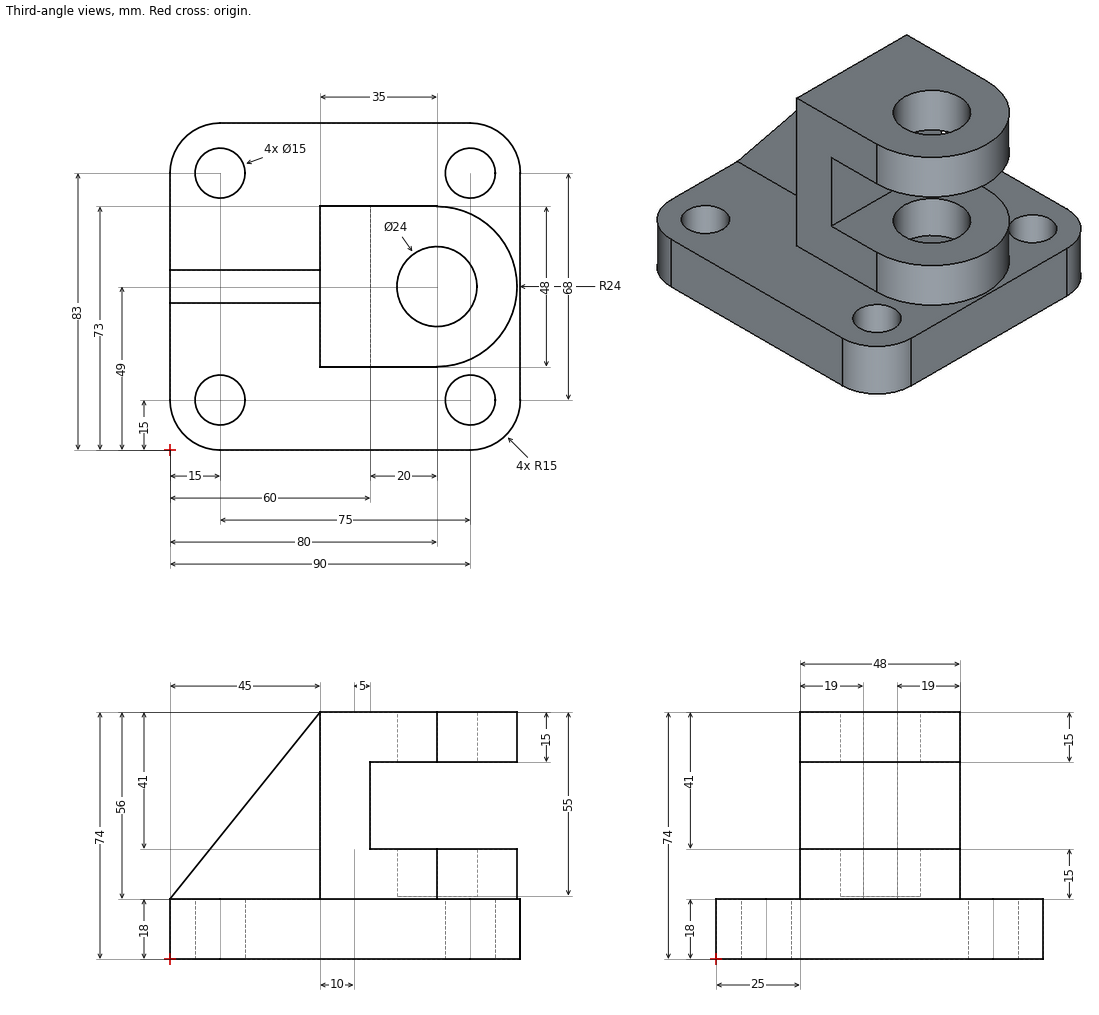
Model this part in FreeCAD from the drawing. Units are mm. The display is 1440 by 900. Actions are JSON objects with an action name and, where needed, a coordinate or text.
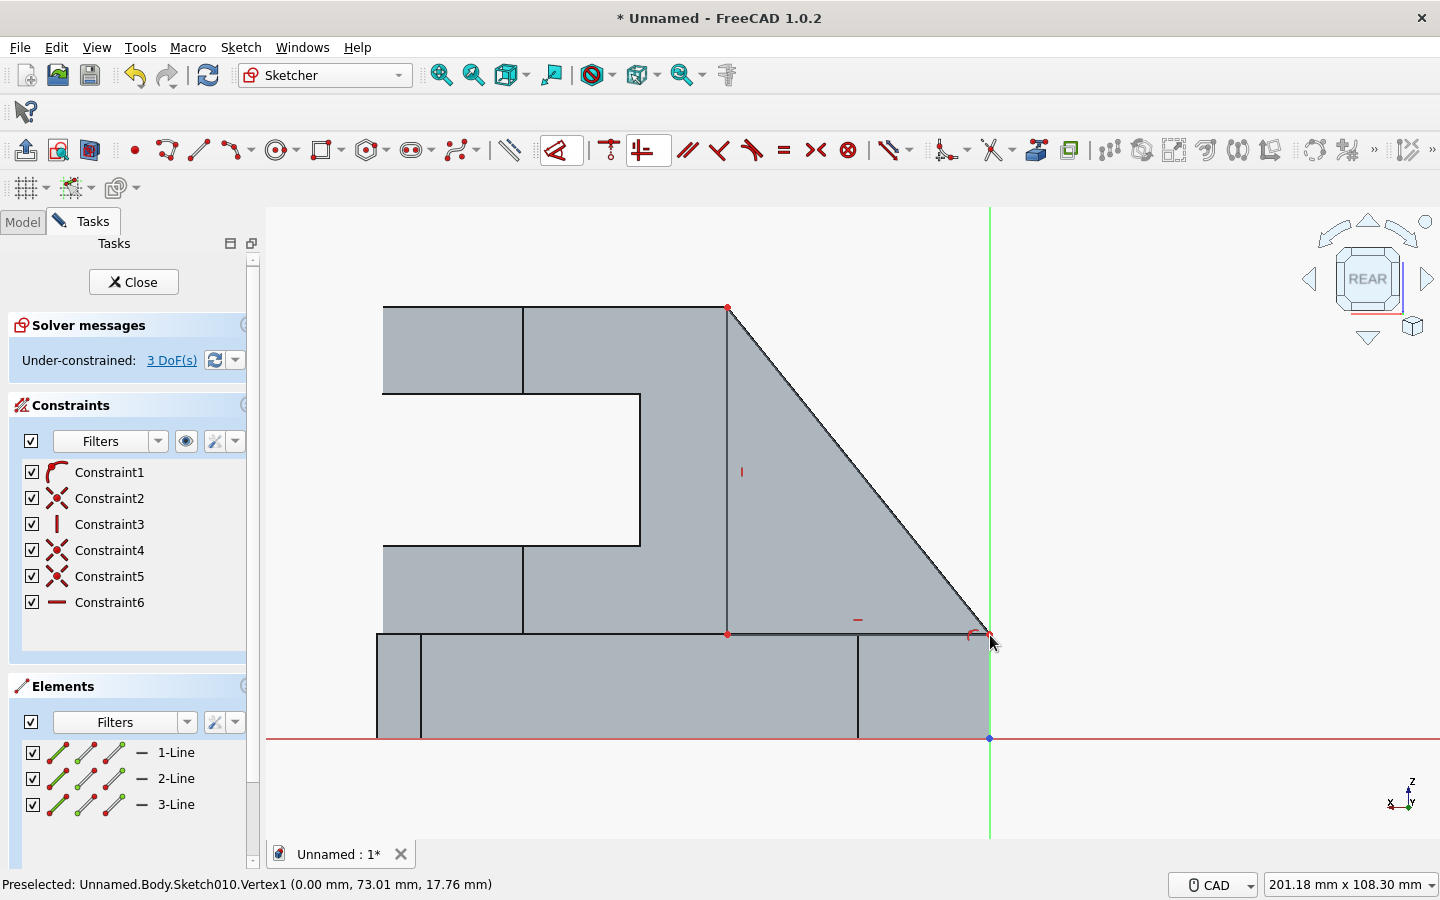
{"action": "left_click", "coordinate": [727, 406]}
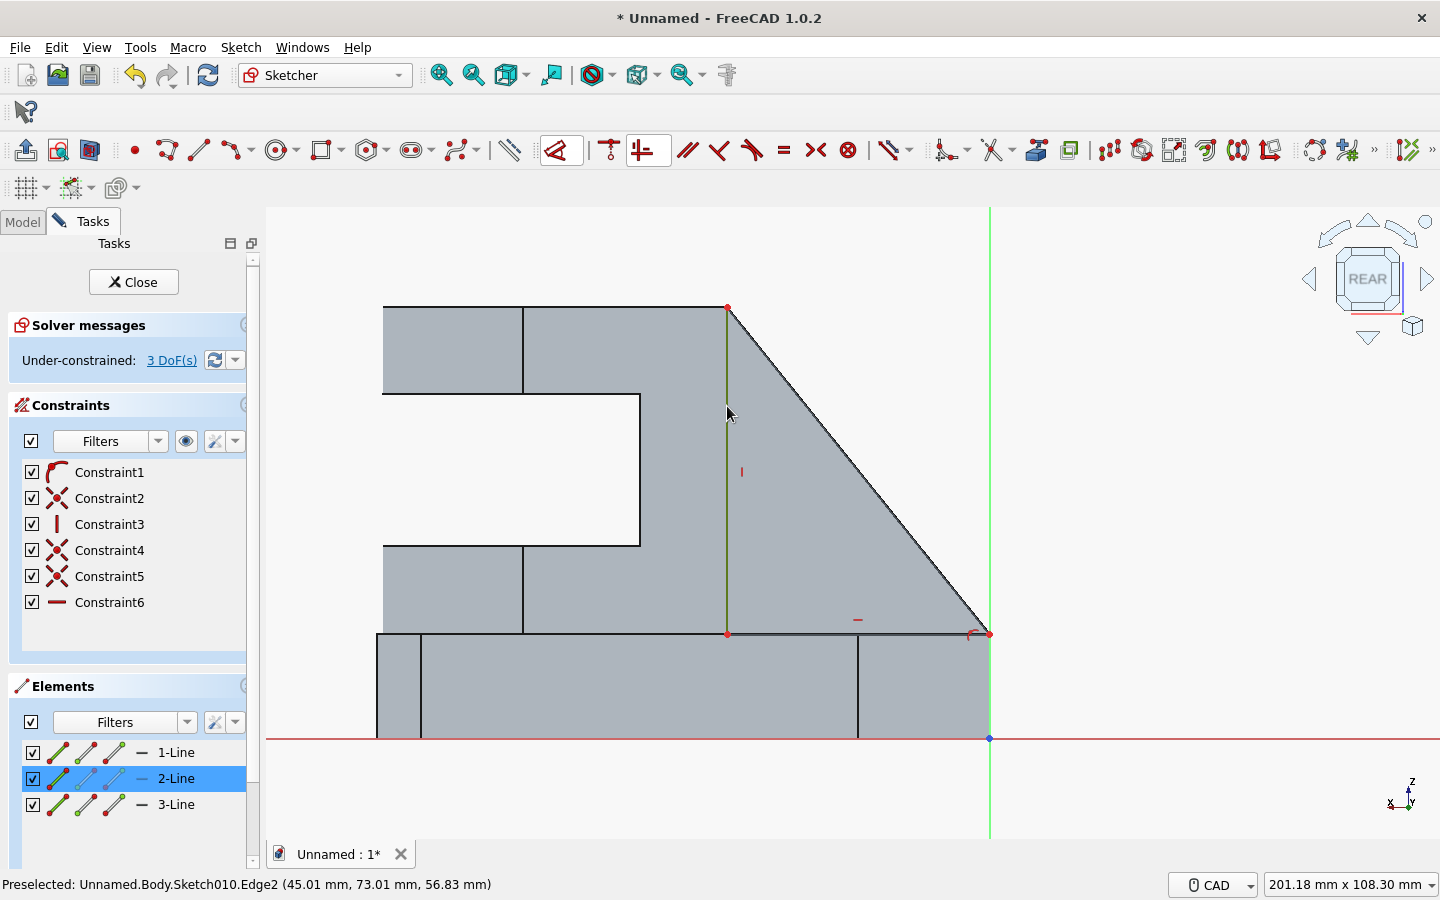
{"action": "left_click", "coordinate": [578, 150]}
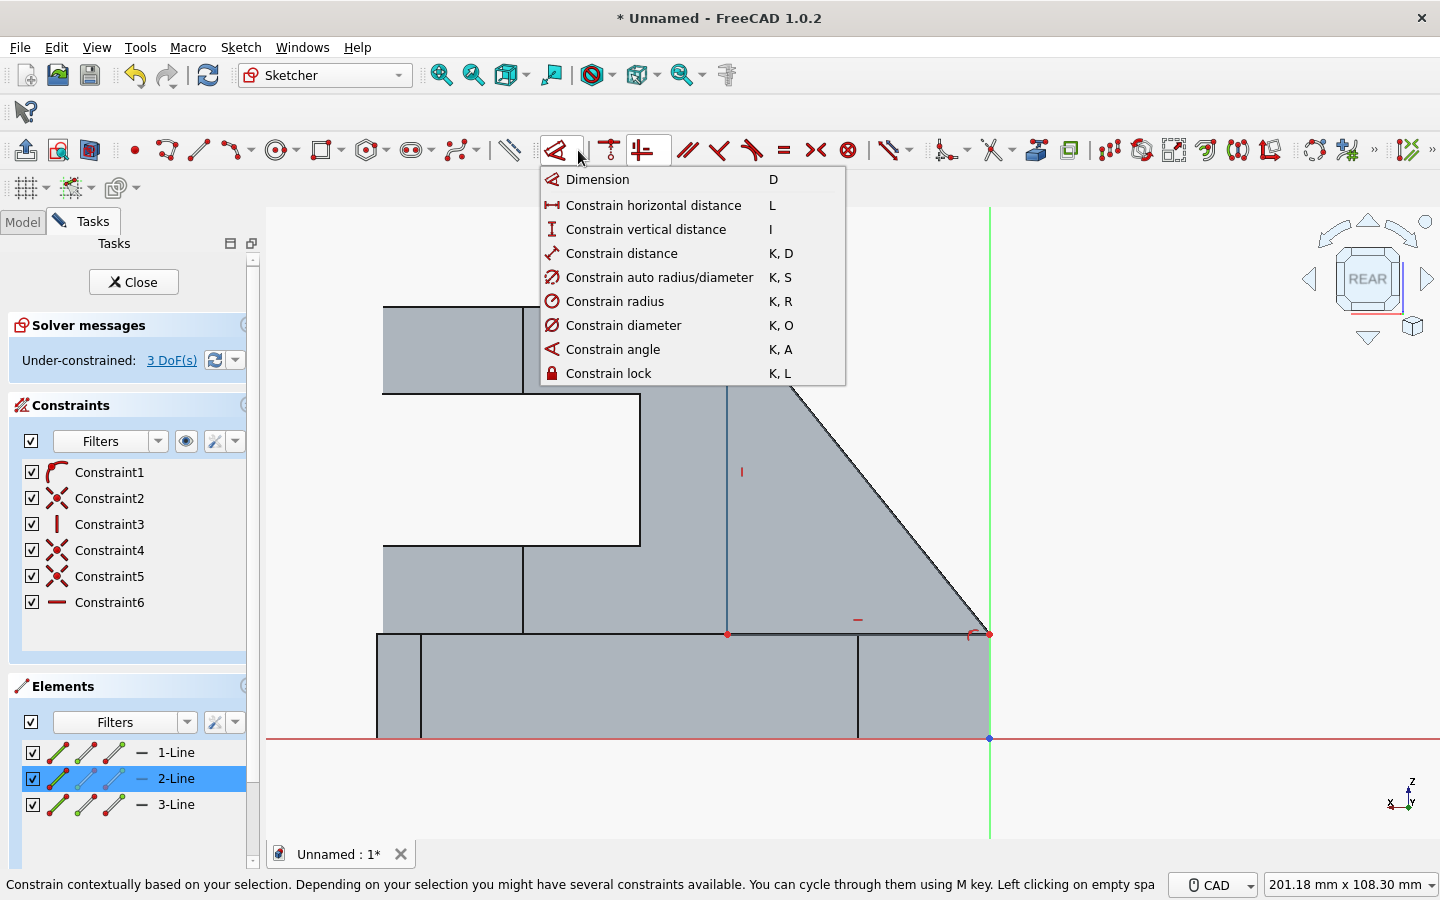
{"action": "left_click", "coordinate": [693, 229]}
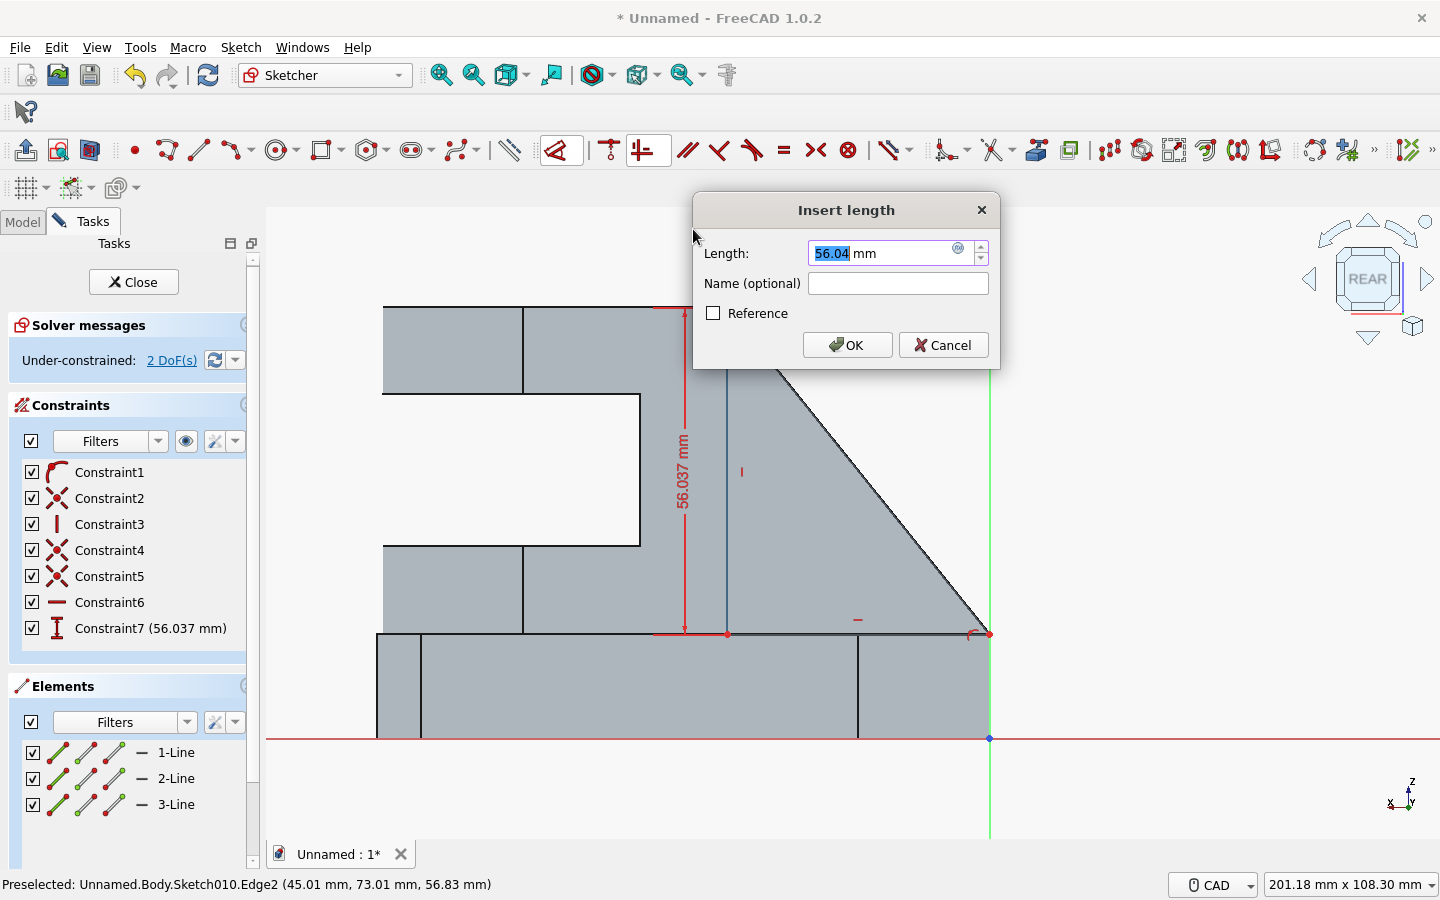
{"action": "type", "text": "56"}
{"action": "key", "text": "Return"}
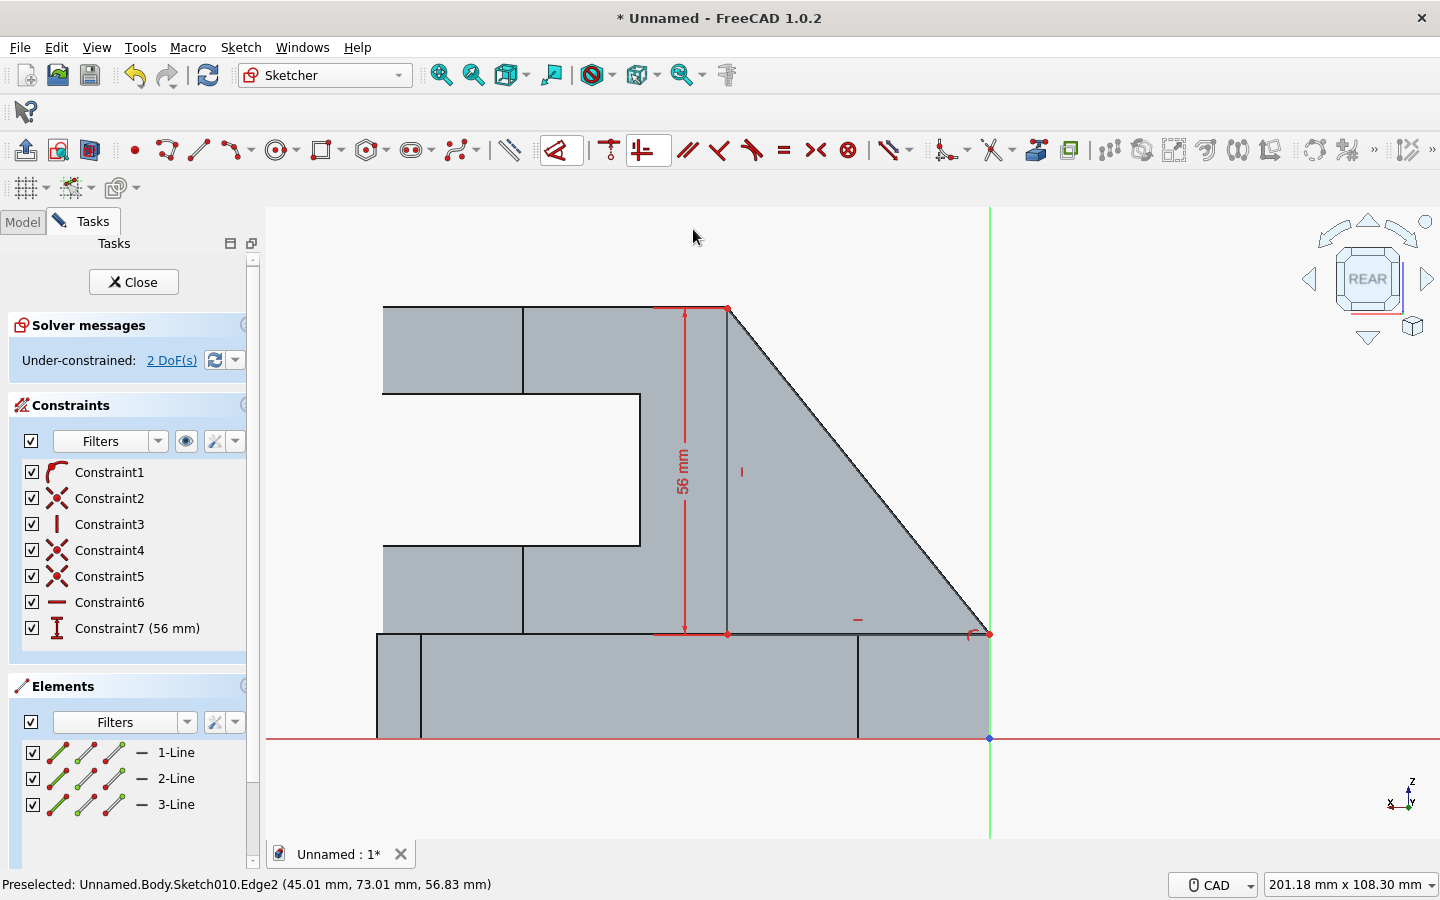
{"action": "left_click", "coordinate": [806, 635]}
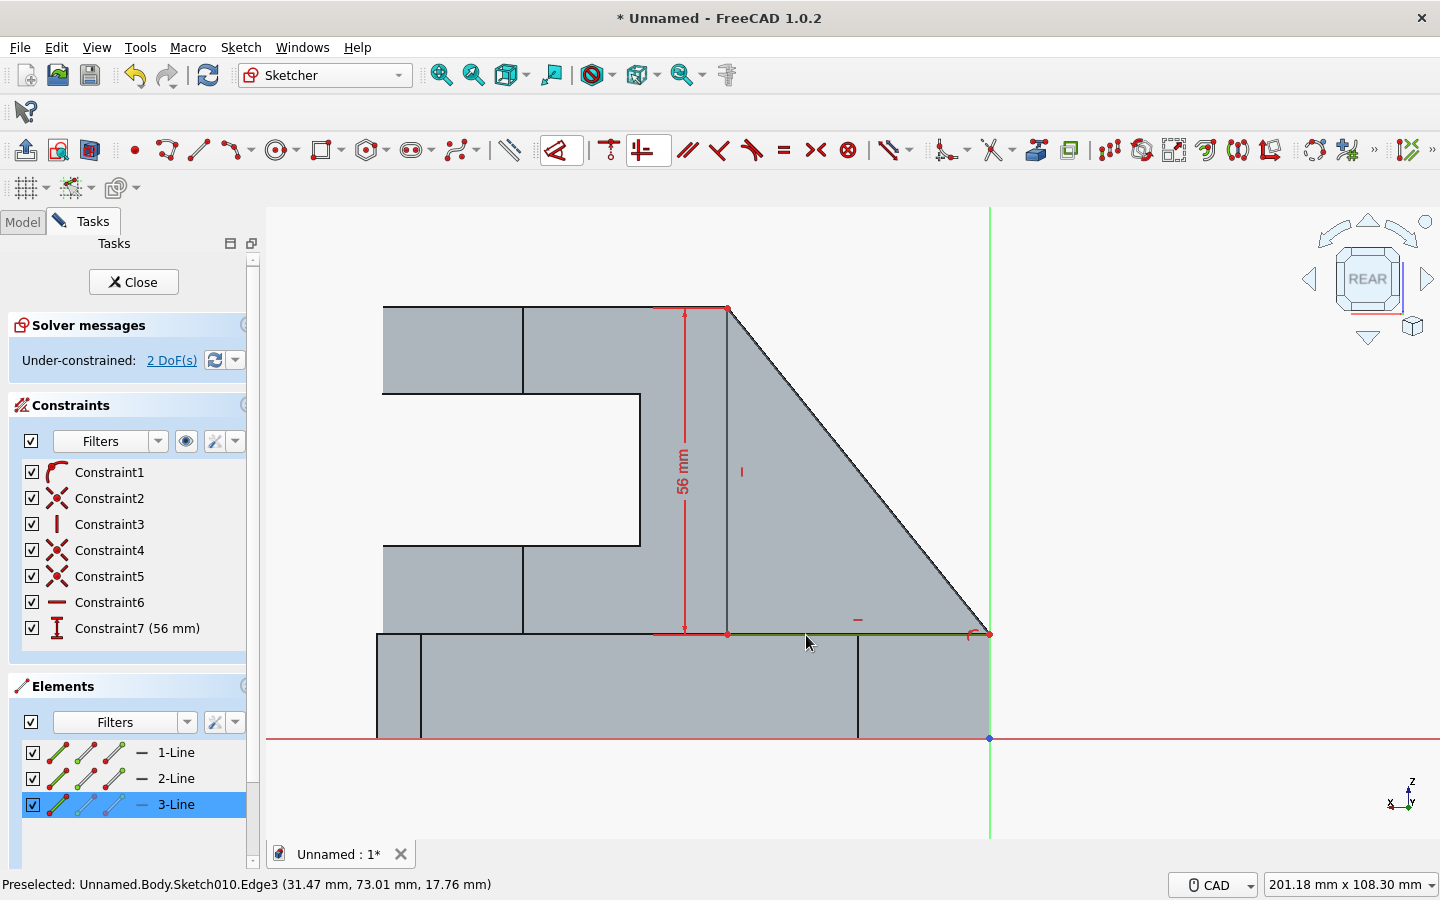
{"action": "left_click", "coordinate": [578, 150]}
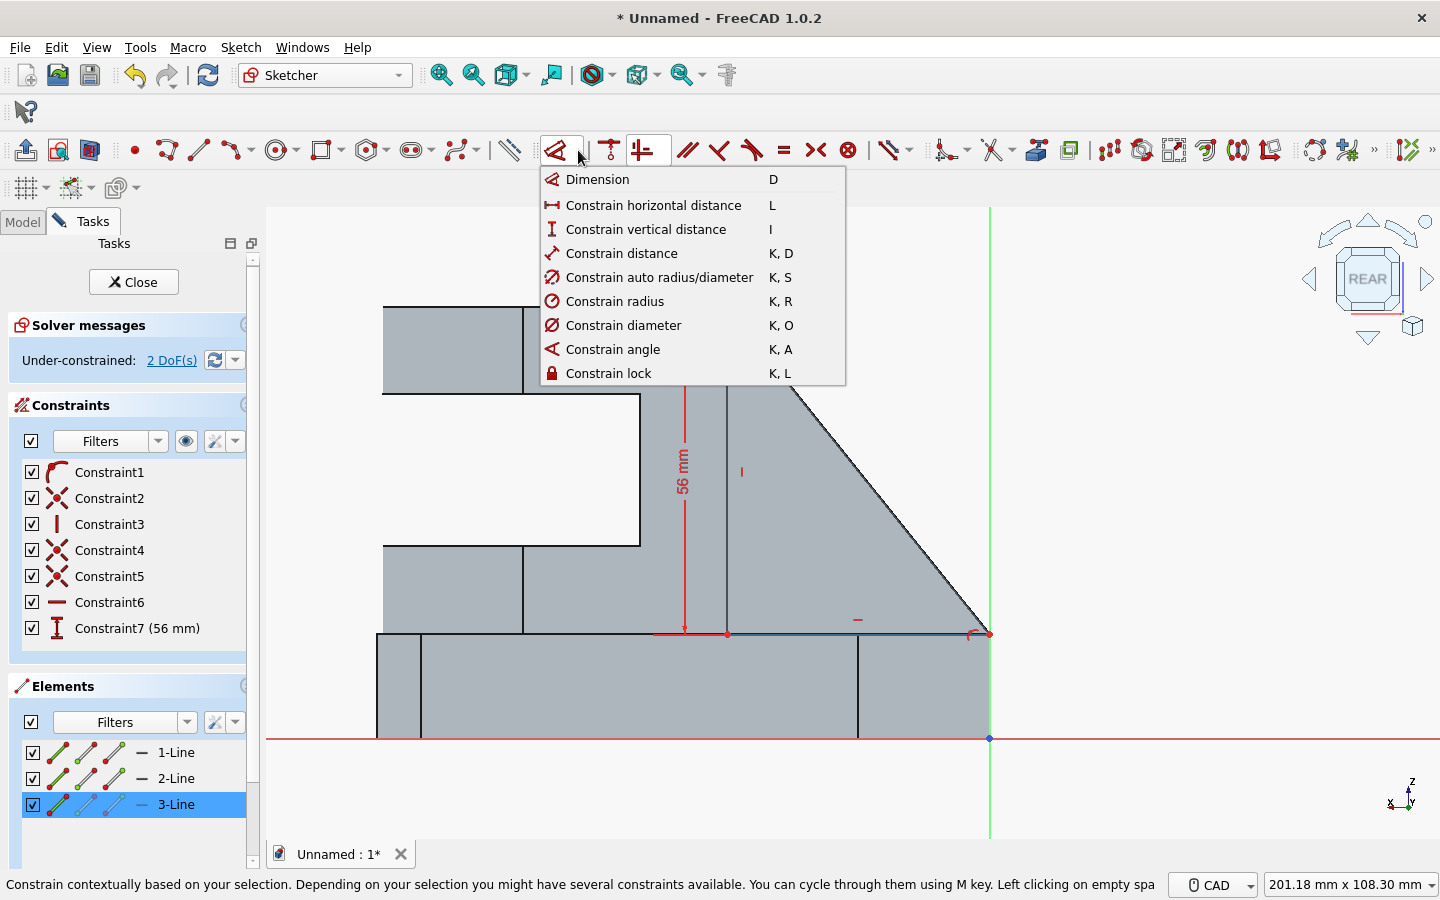
{"action": "left_click", "coordinate": [693, 205]}